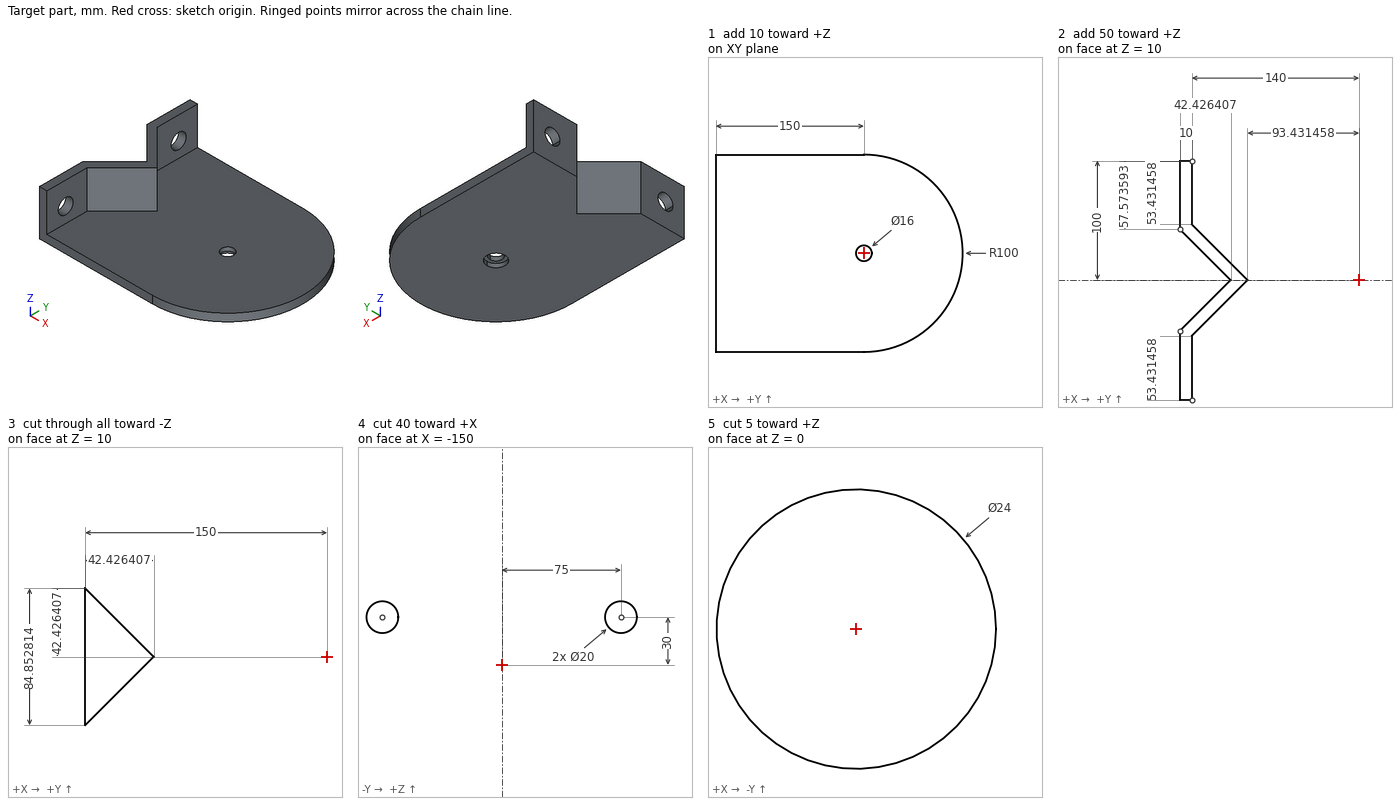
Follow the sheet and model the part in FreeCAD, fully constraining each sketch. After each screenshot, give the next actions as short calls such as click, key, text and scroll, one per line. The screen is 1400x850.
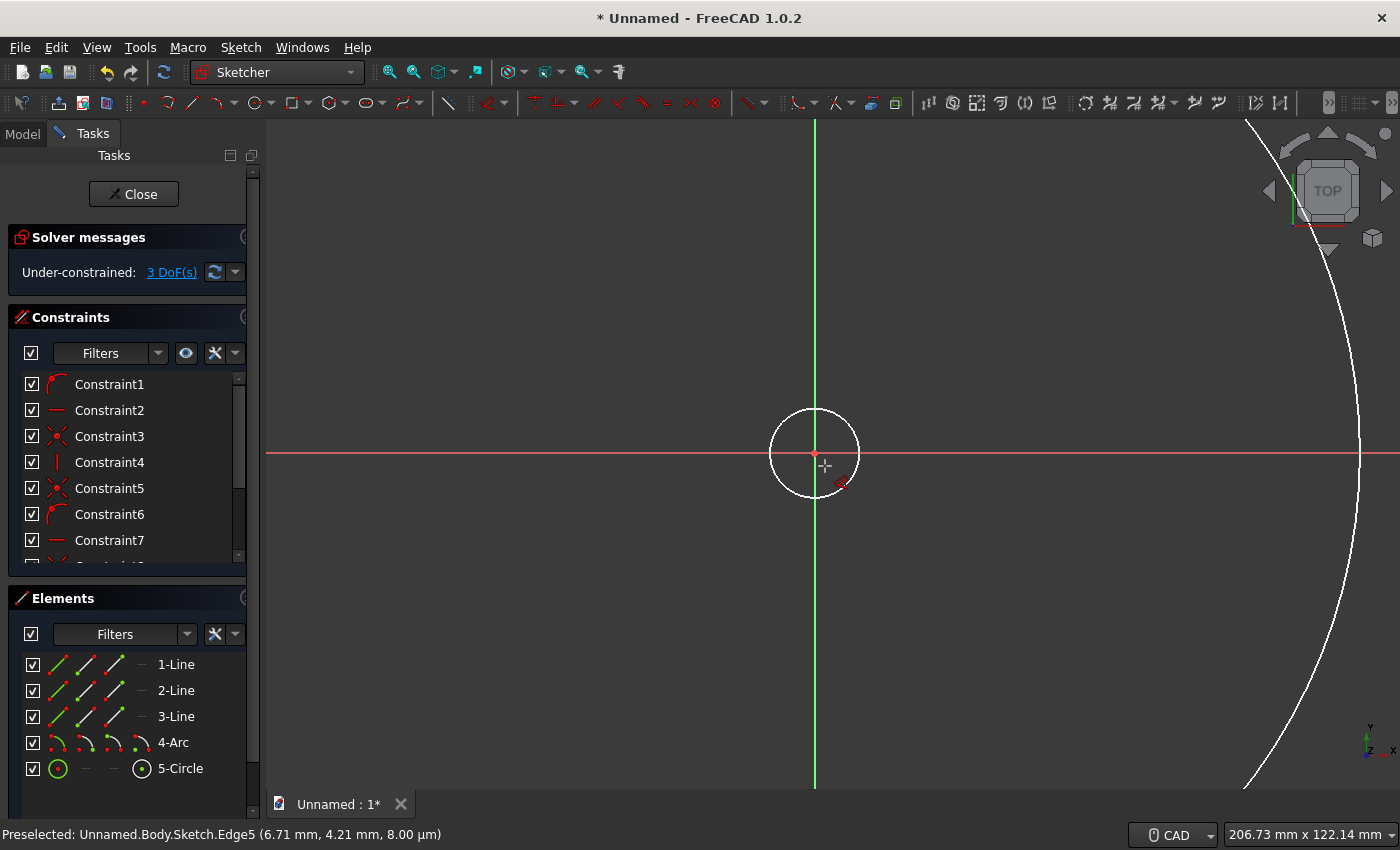
scroll(815, 454, down, 5)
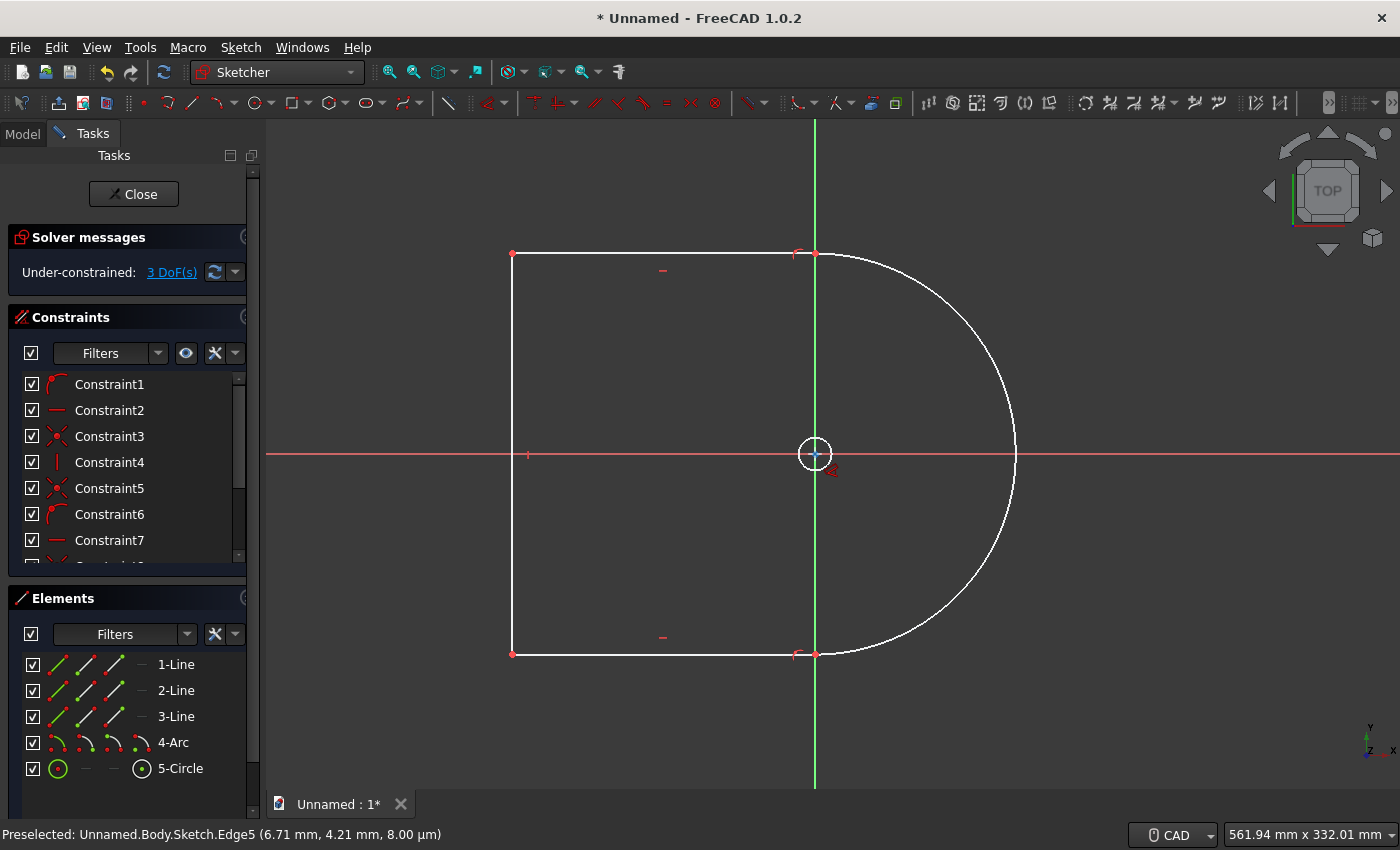
click(977, 572)
click(1003, 591)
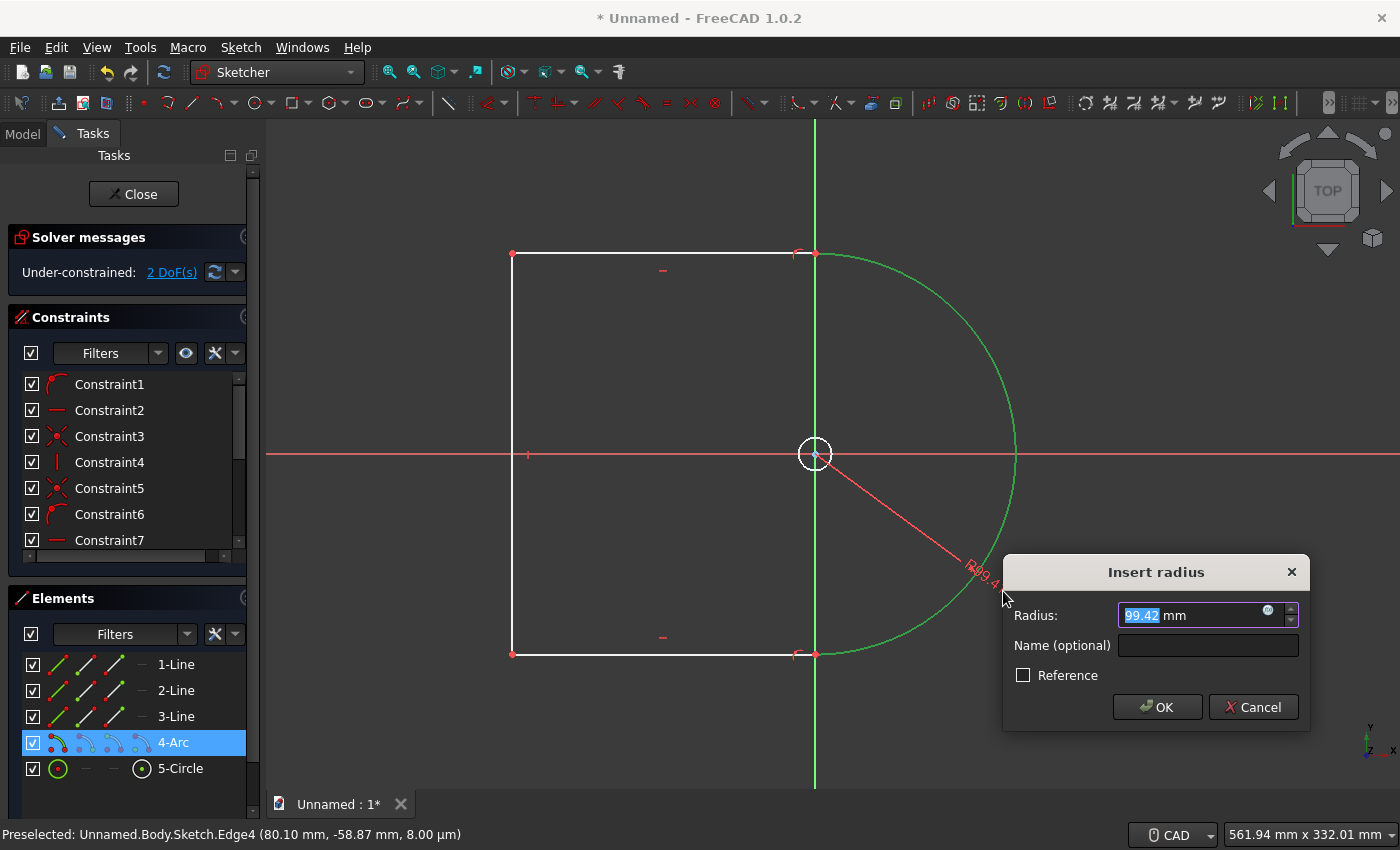
text(100)
key(Return)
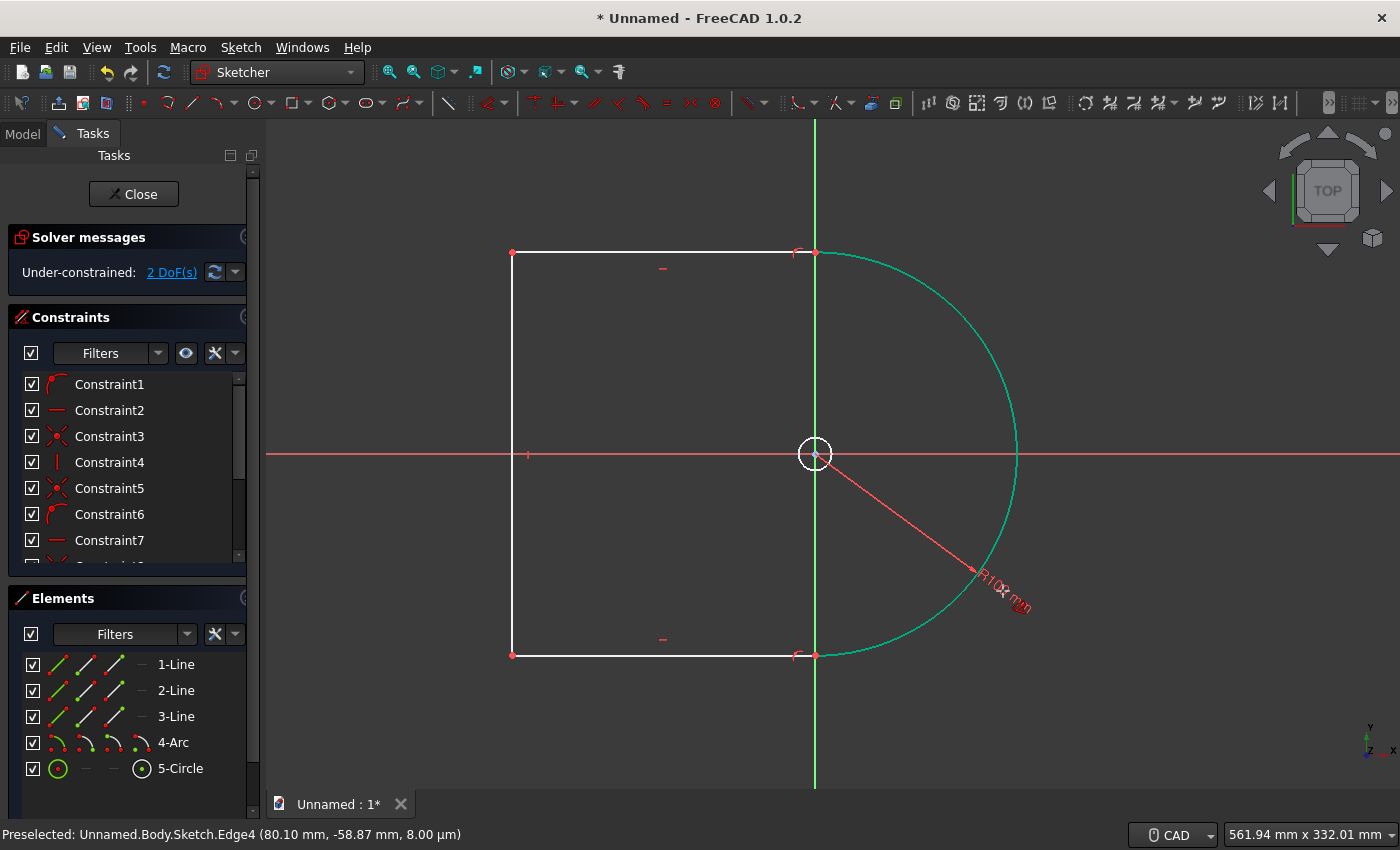
scroll(827, 442, up, 2)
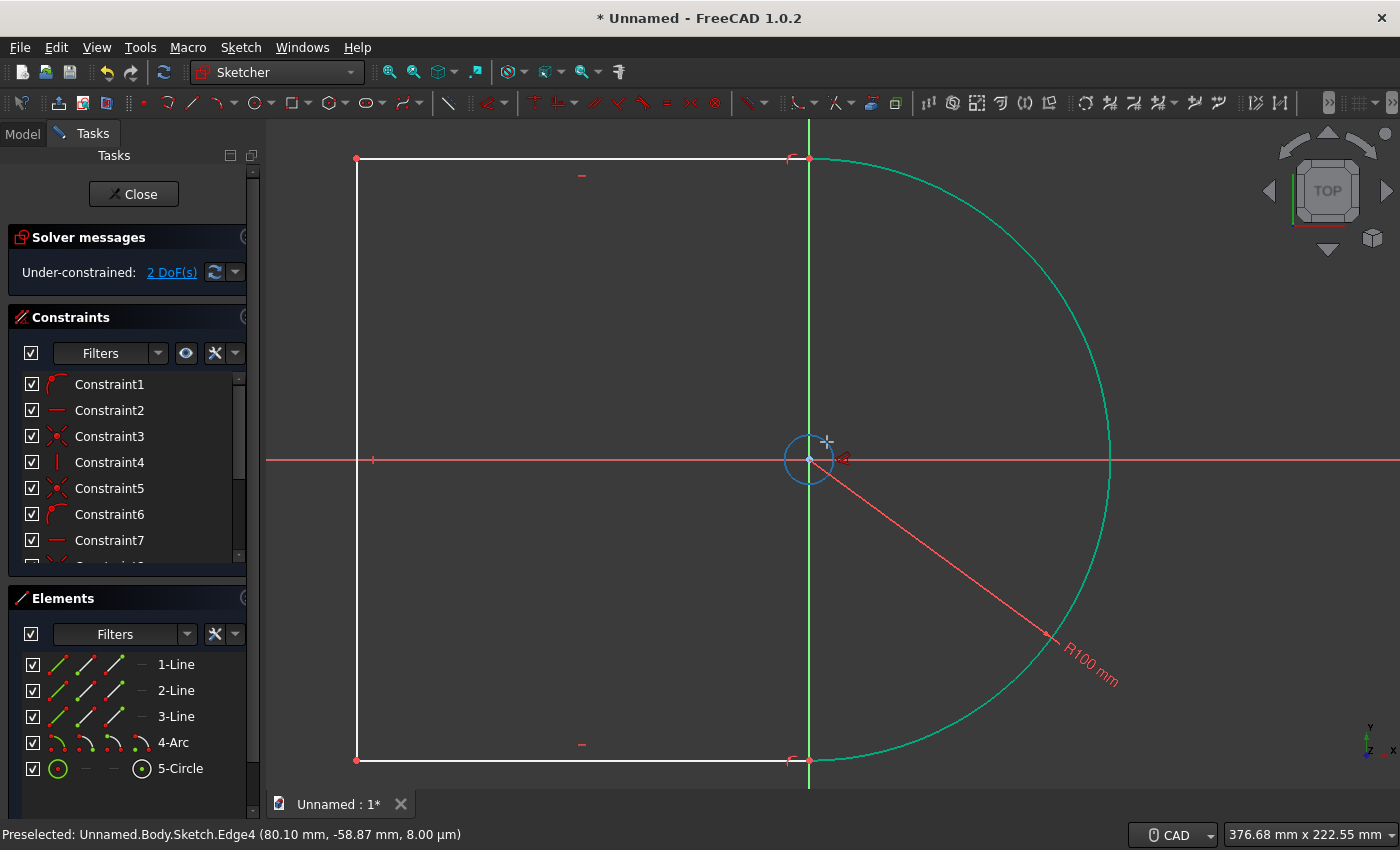
click(826, 442)
click(848, 419)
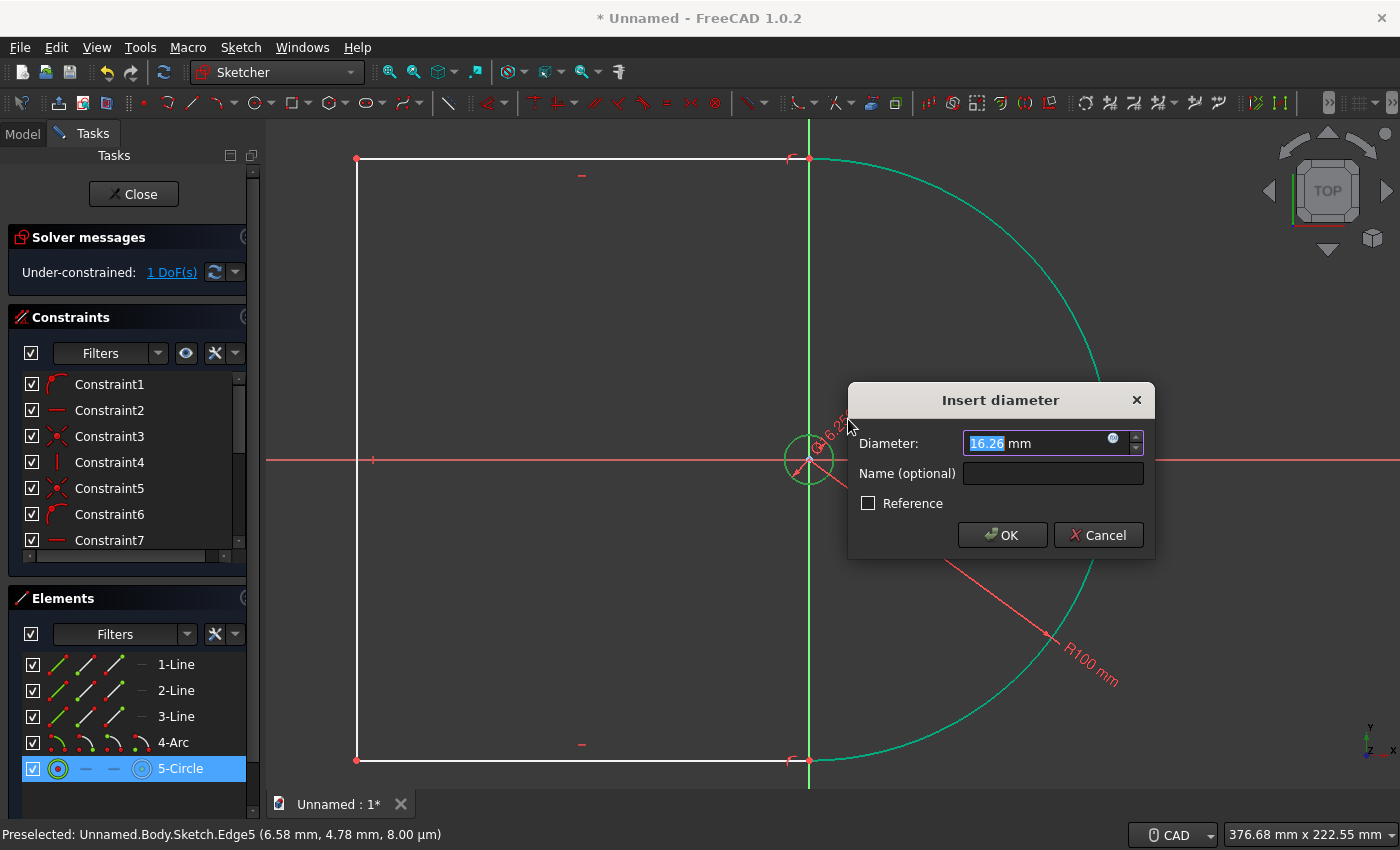
text(16)
key(Return)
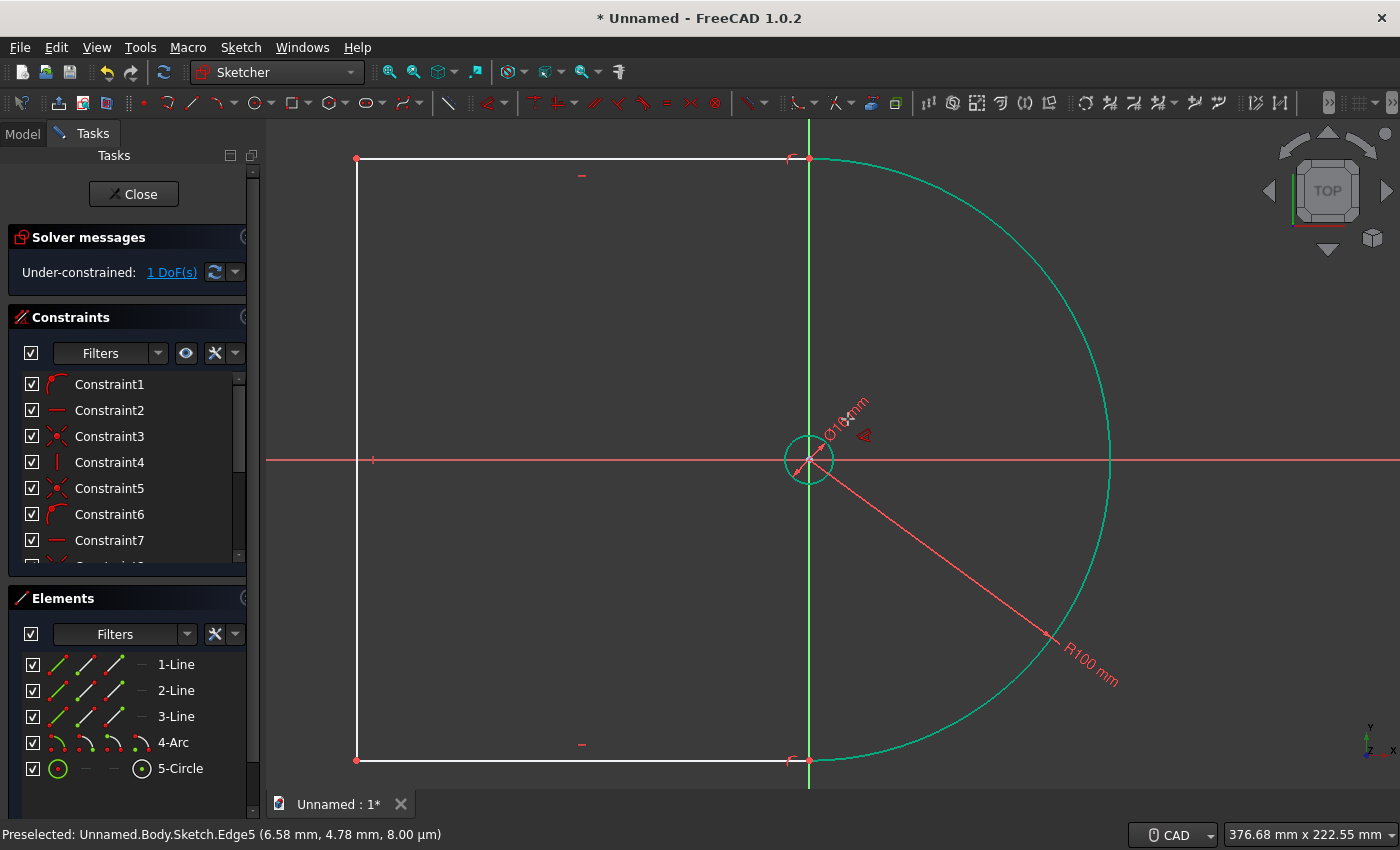
click(673, 159)
click(583, 193)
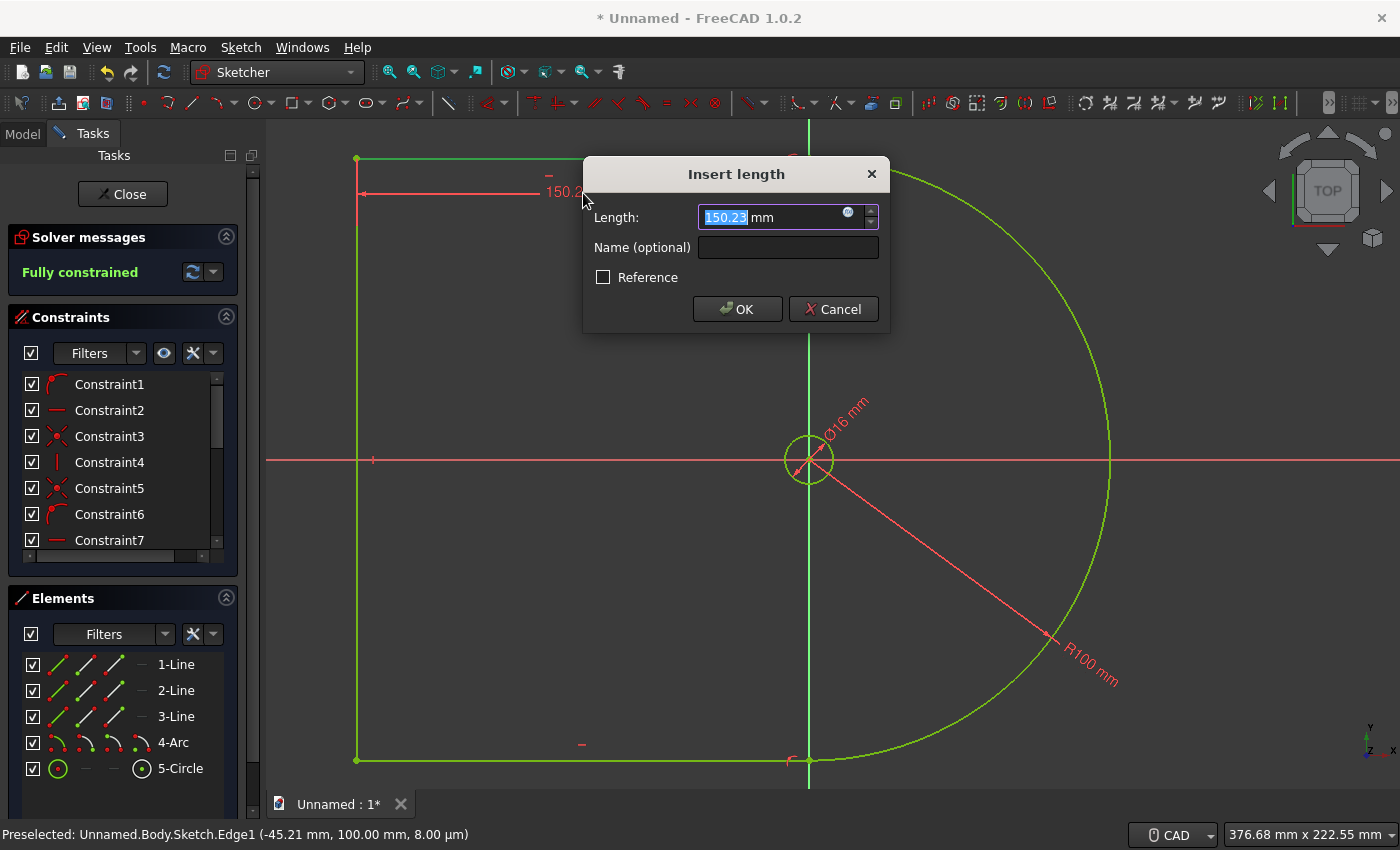
text(150)
key(Return)
key(Escape)